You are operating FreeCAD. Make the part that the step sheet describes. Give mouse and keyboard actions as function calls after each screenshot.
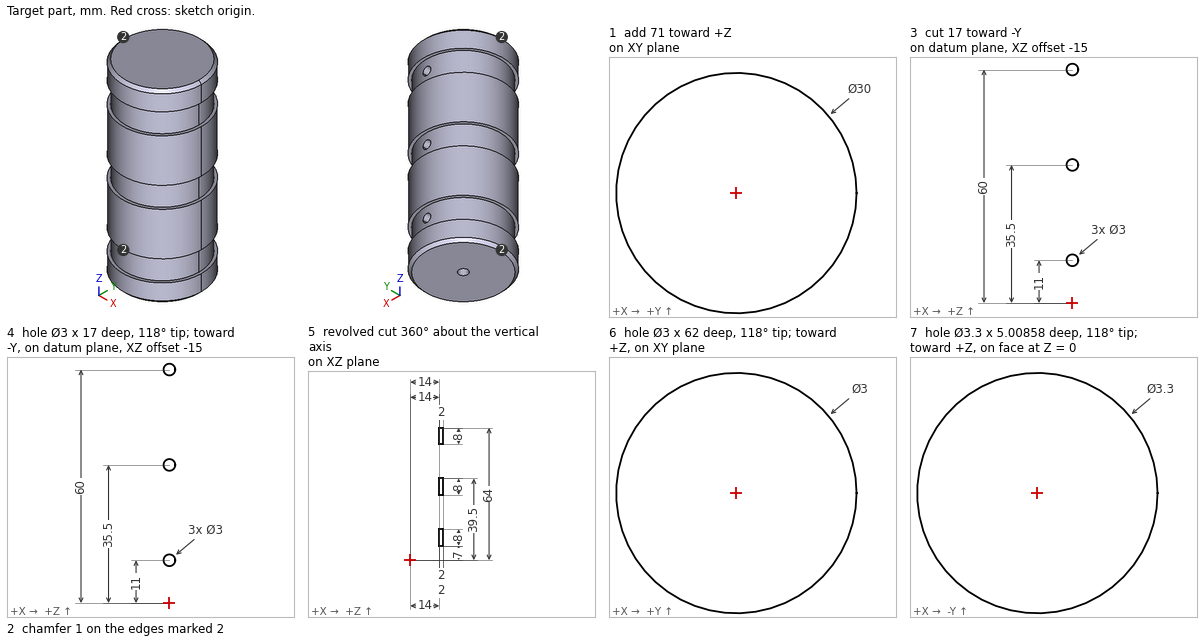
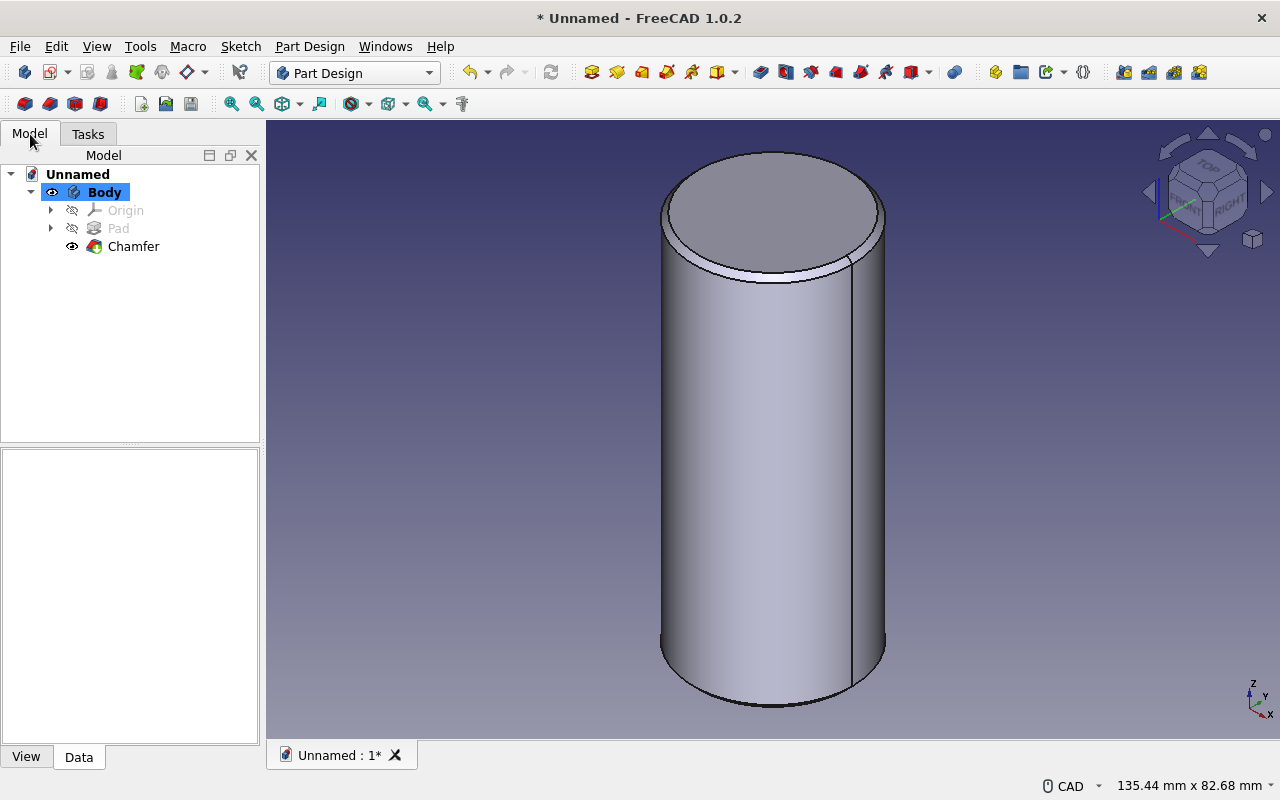
click(51, 210)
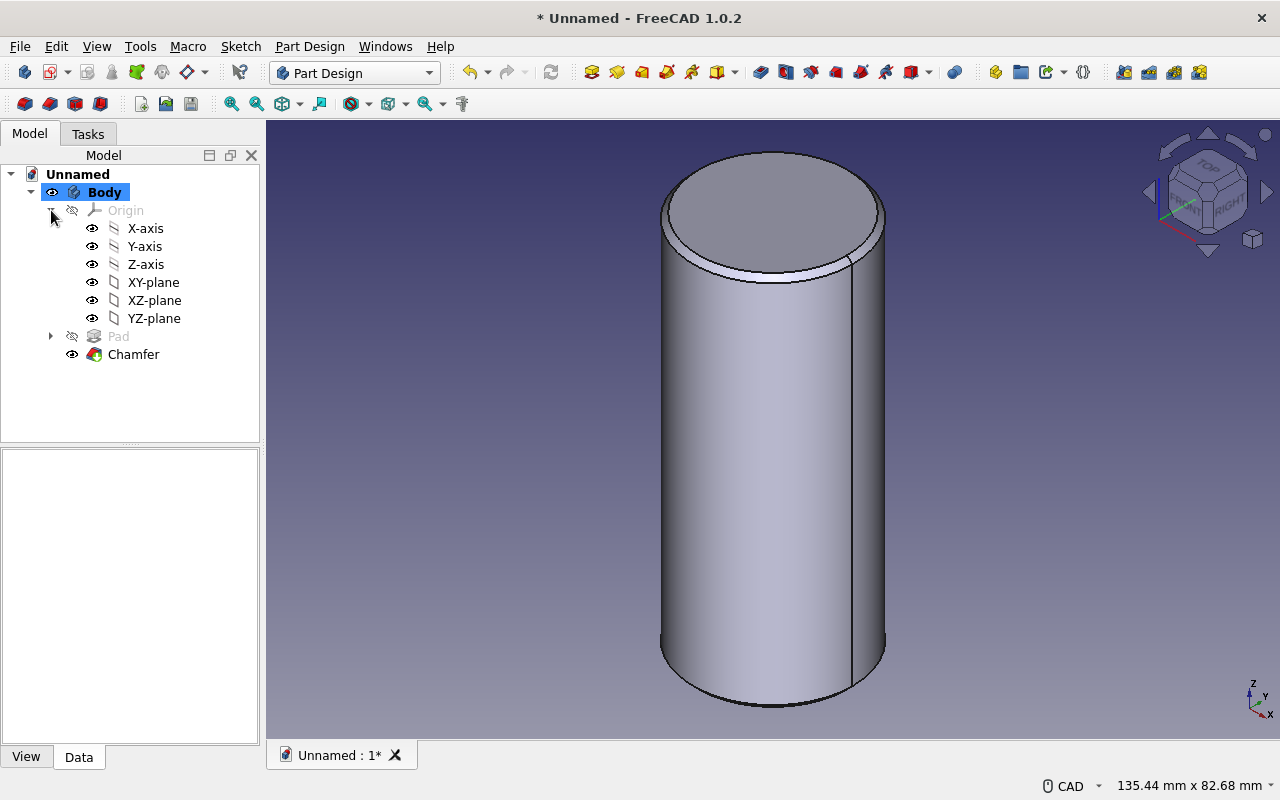
click(137, 300)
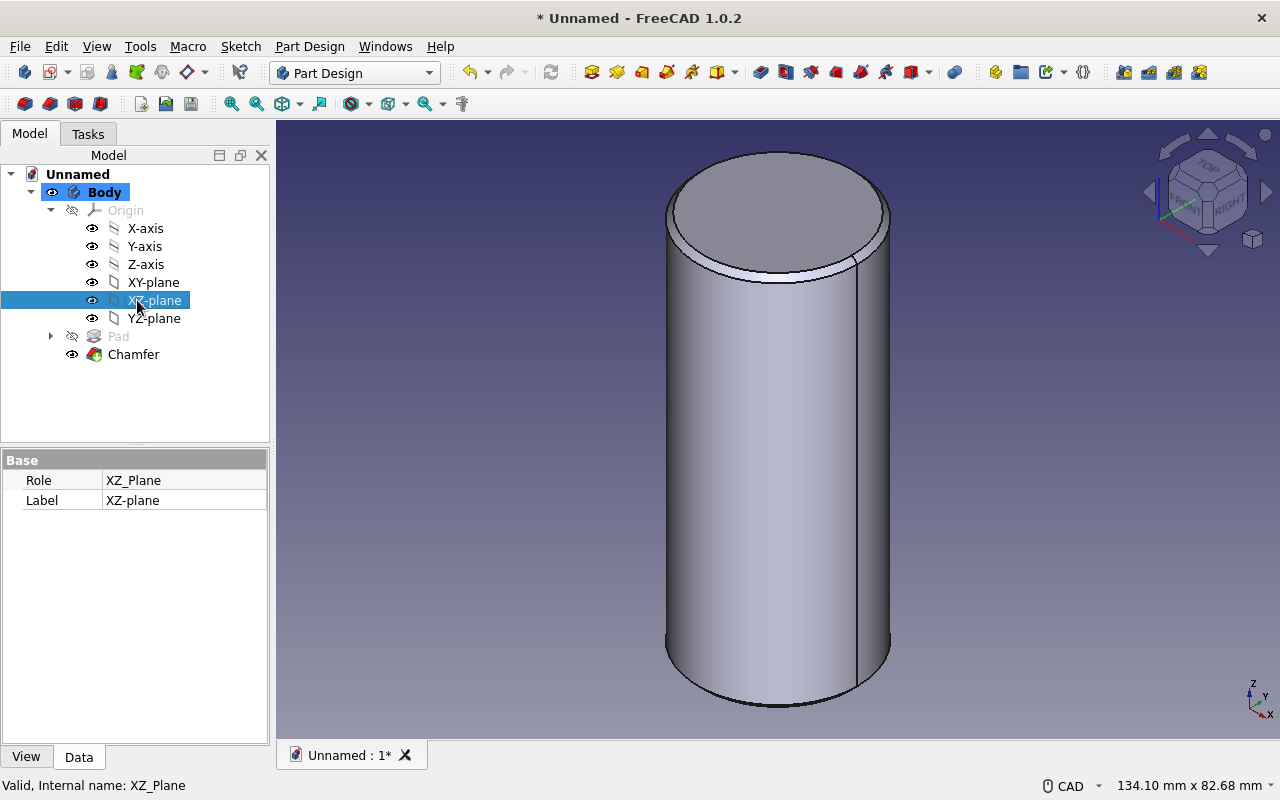
click(186, 72)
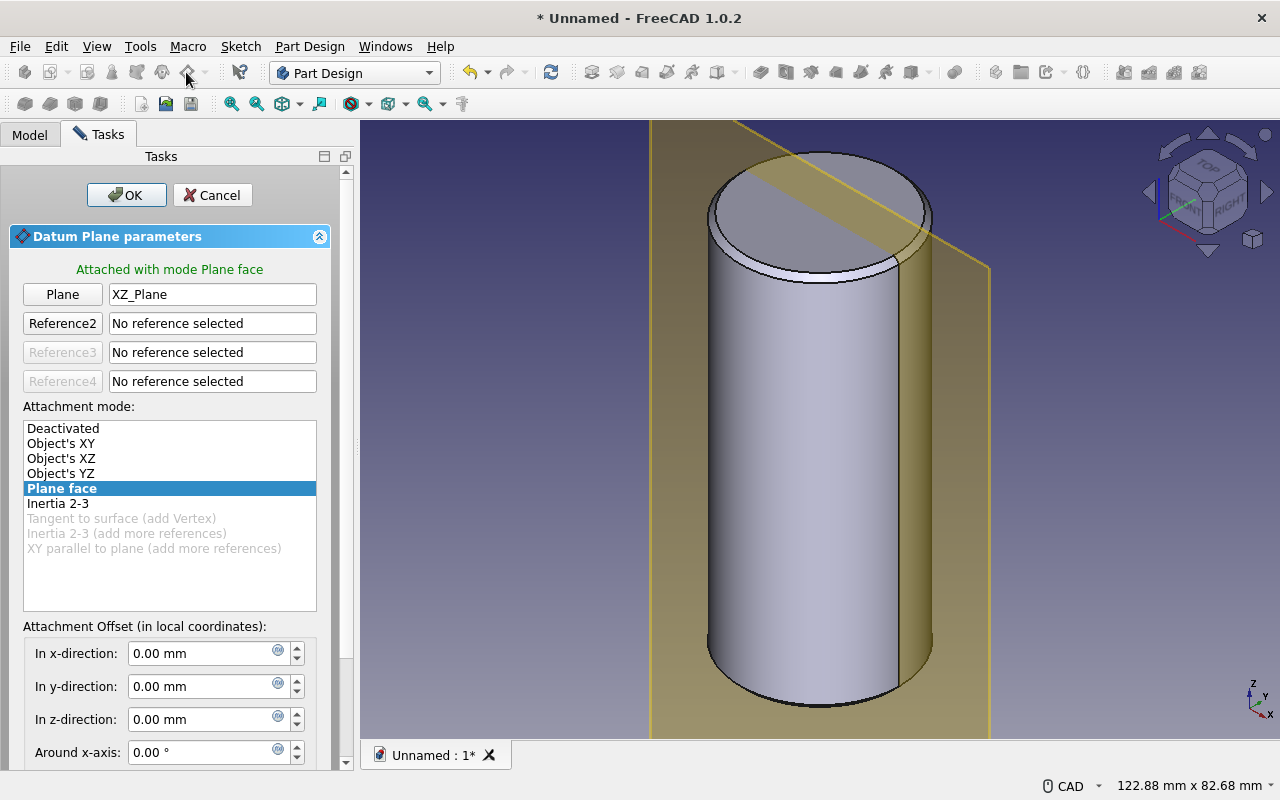
triple_click(210, 720)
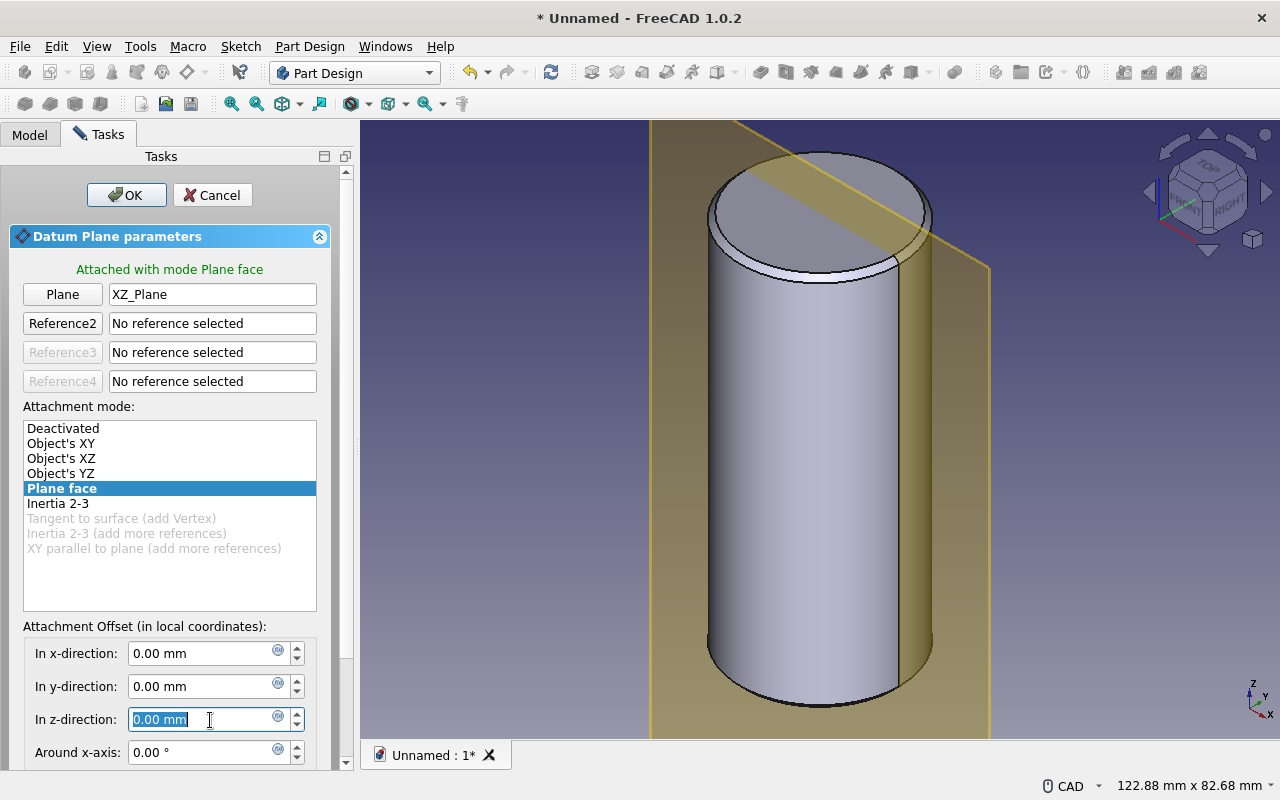
text(-15)
key(Tab)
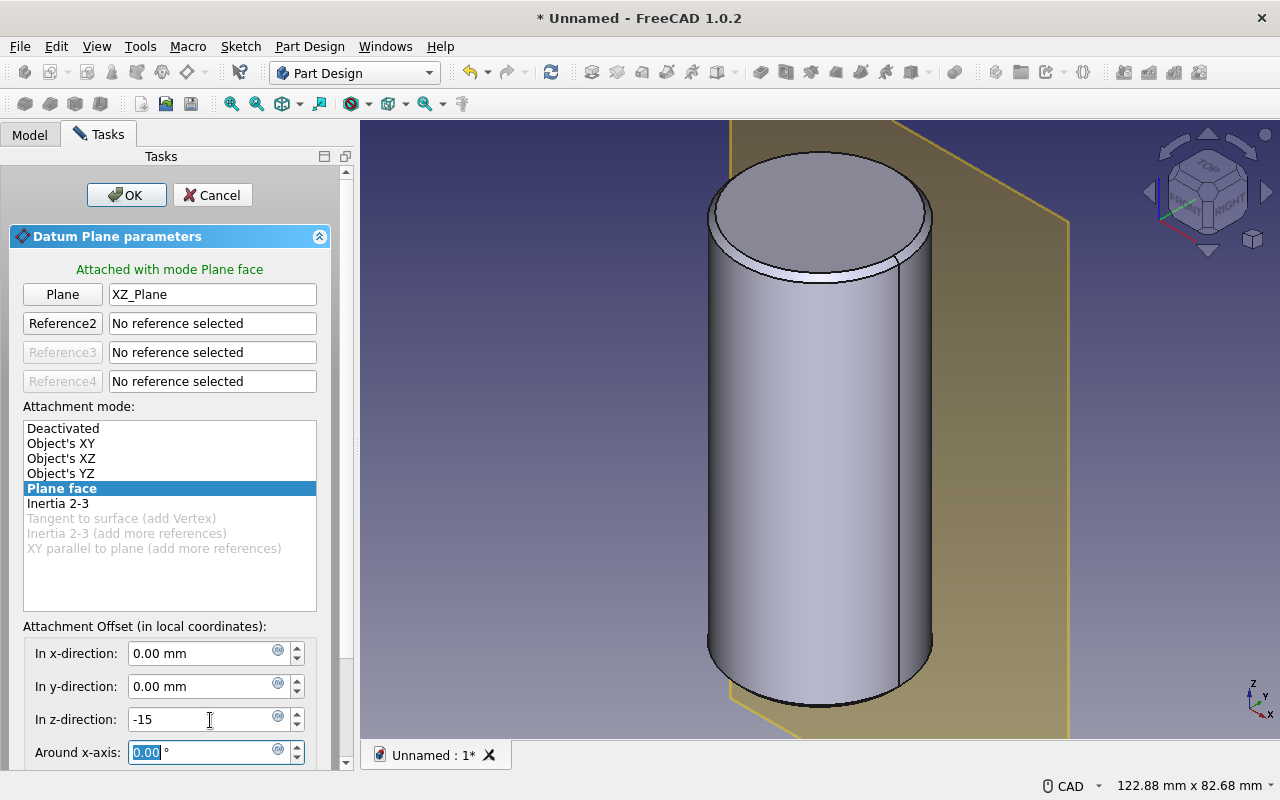
click(127, 195)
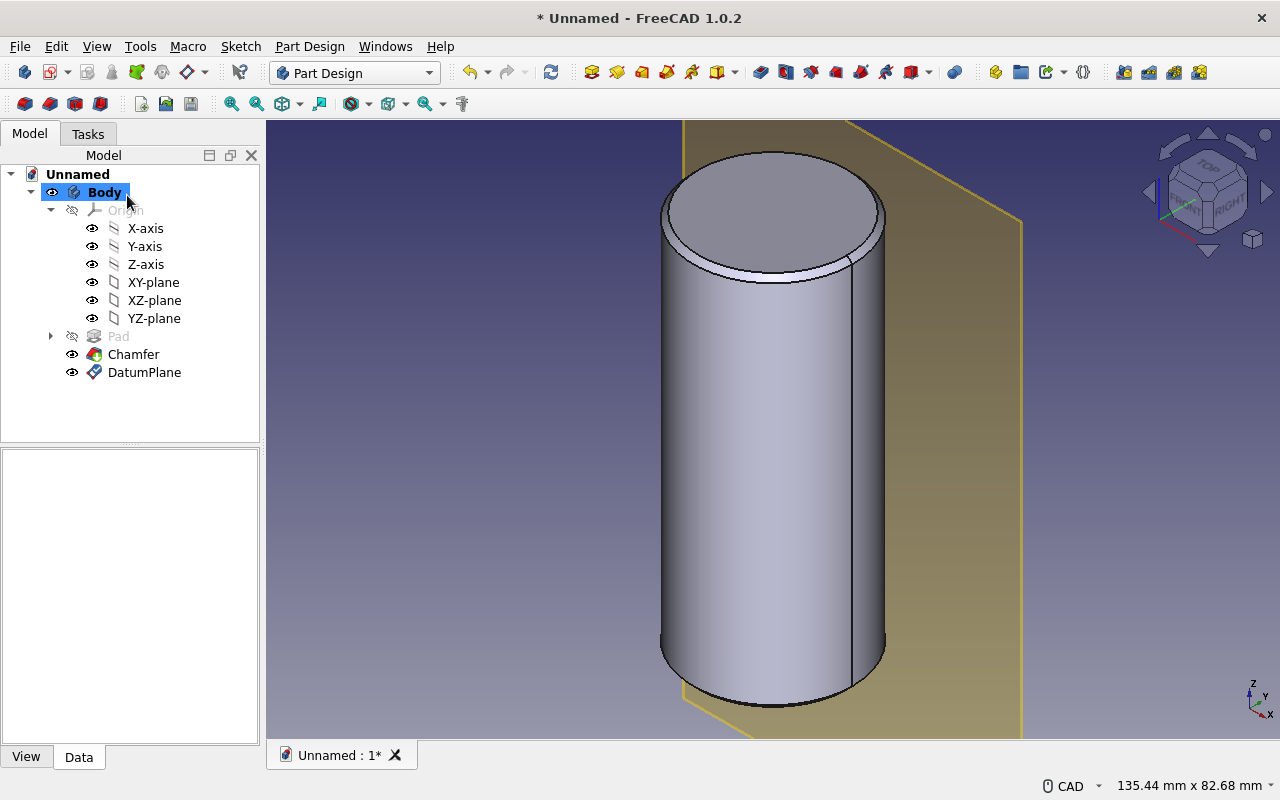
click(117, 372)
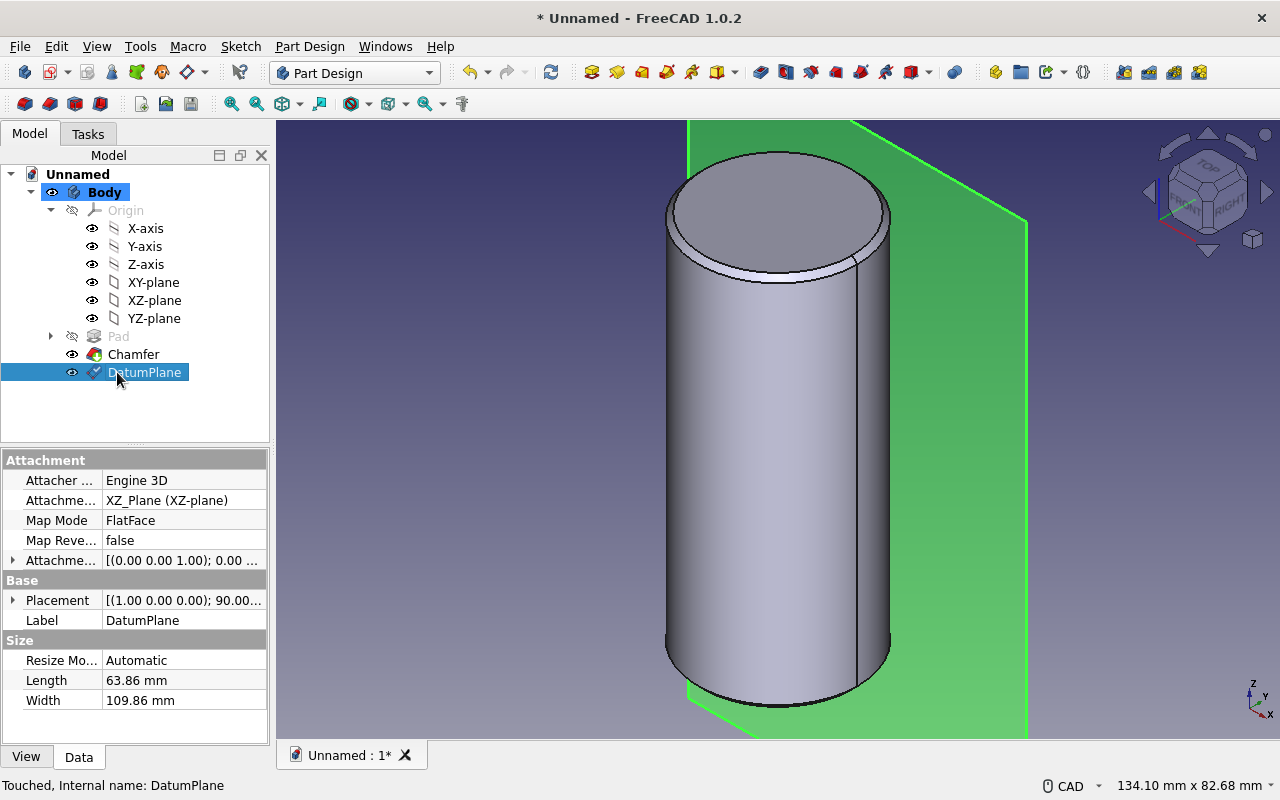
click(50, 72)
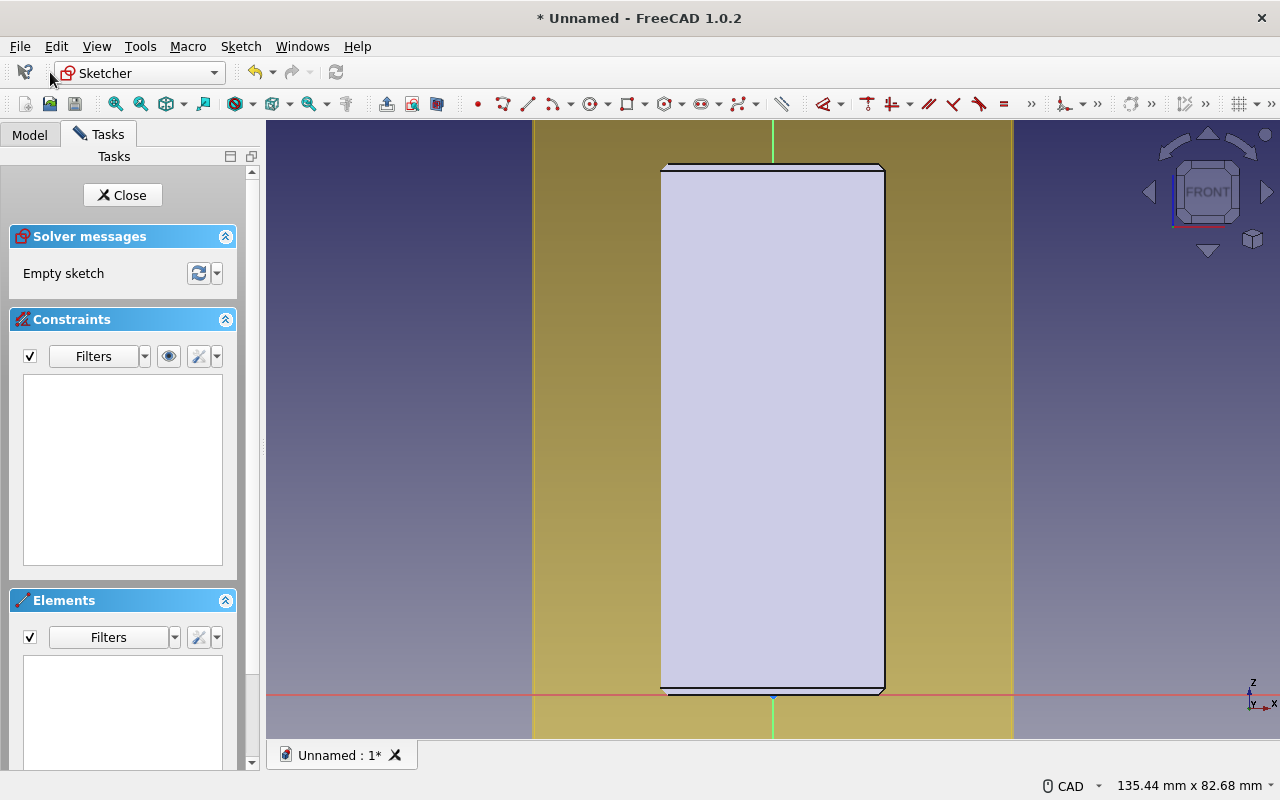
click(437, 104)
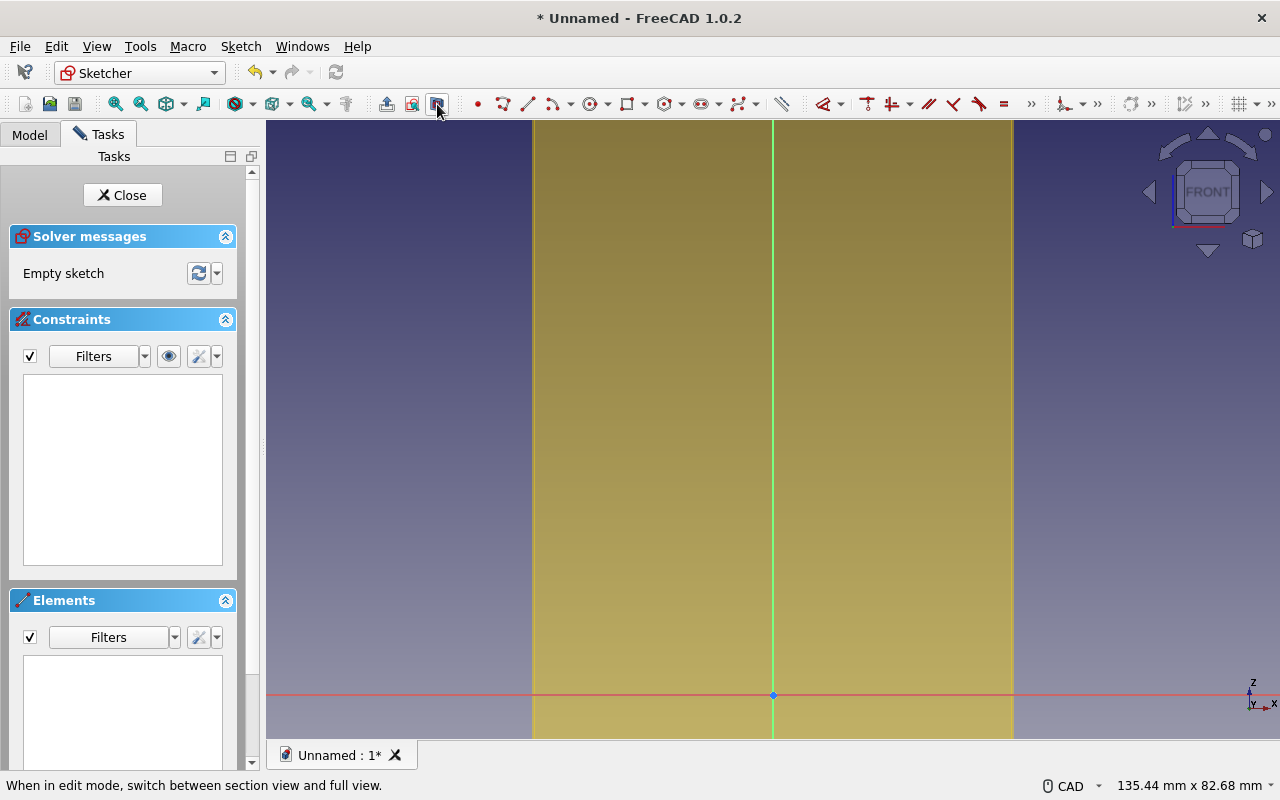
scroll(395, 269, down, 1)